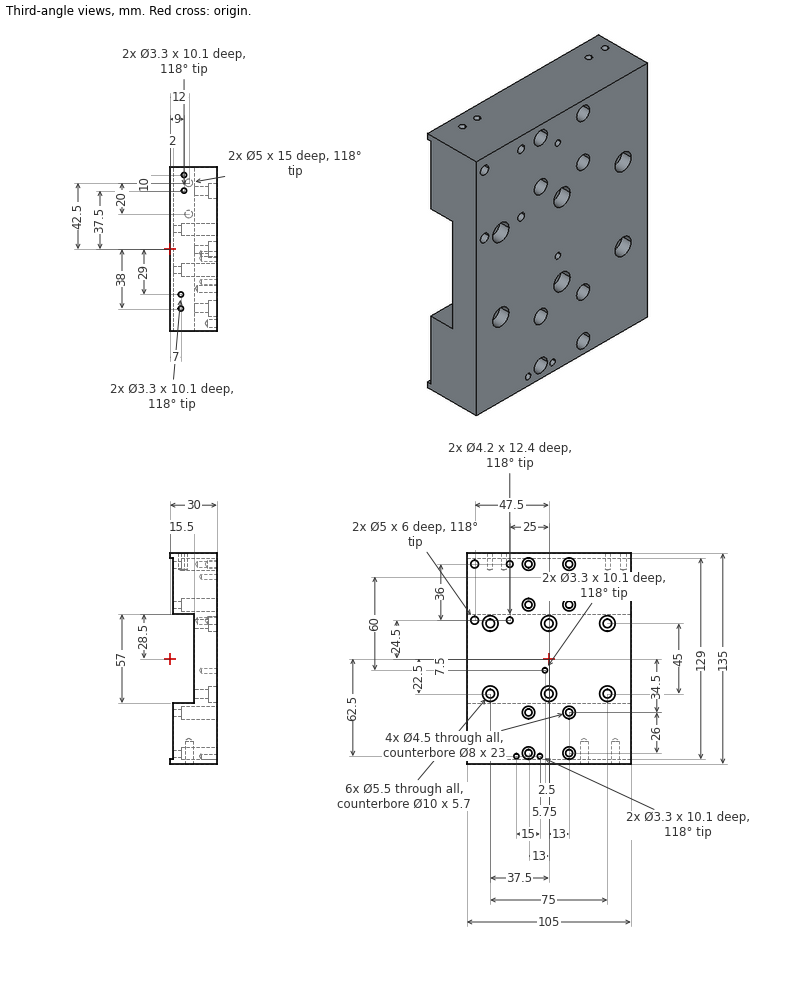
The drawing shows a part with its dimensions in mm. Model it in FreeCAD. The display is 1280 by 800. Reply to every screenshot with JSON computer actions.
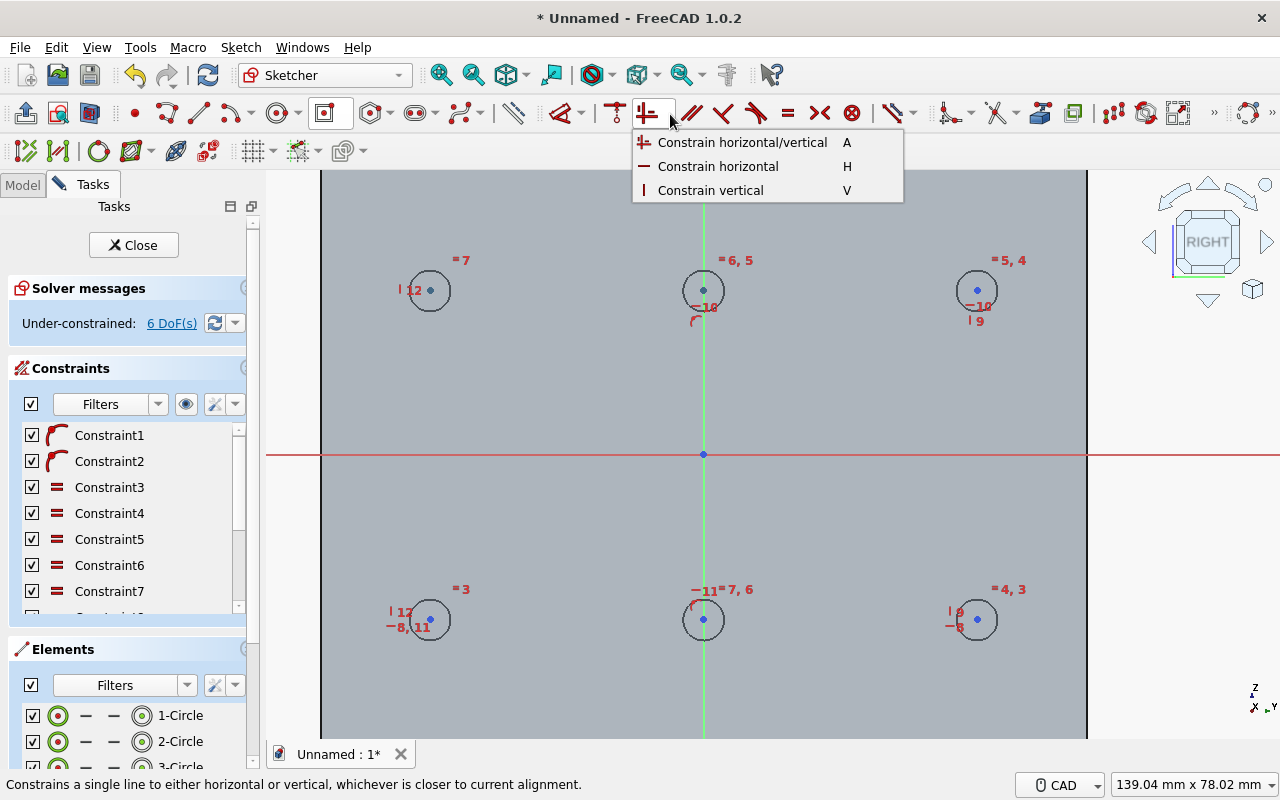
{"action": "left_click", "coordinate": [768, 166]}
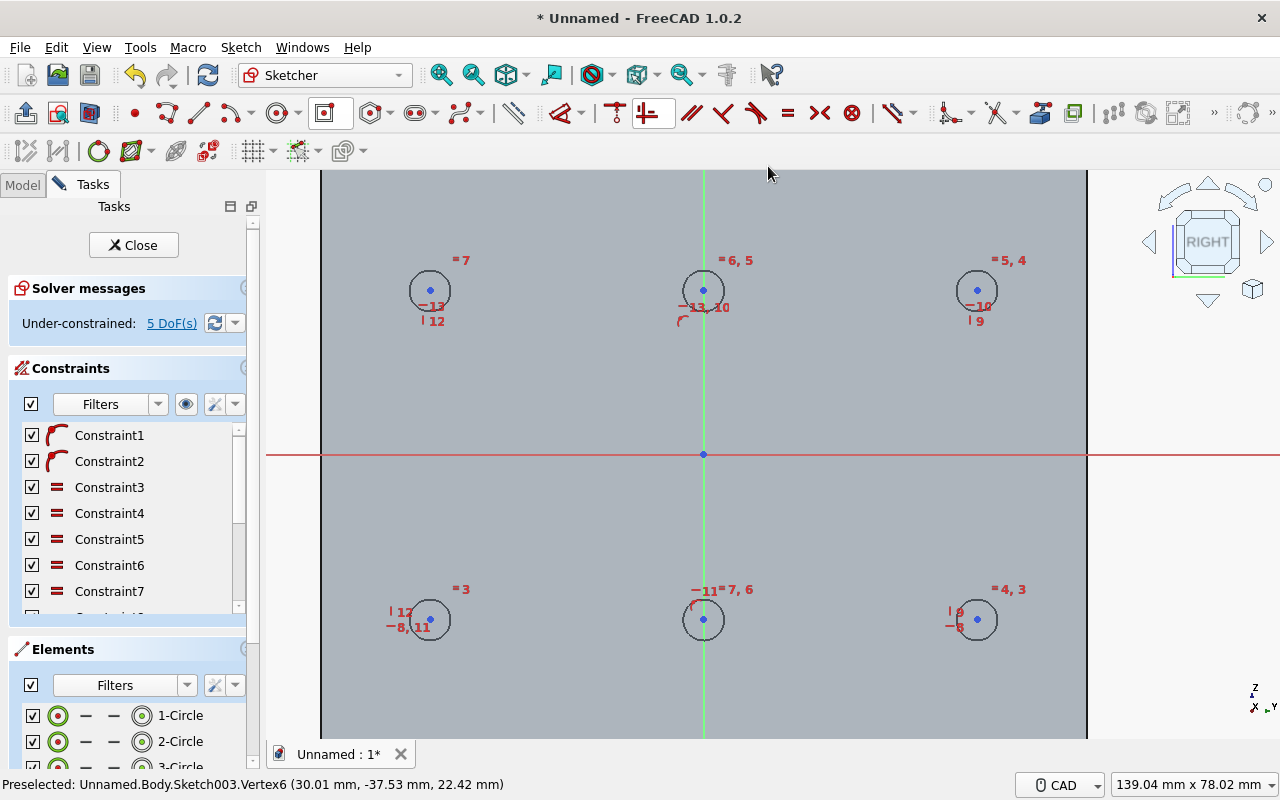
{"action": "left_click", "coordinate": [560, 114]}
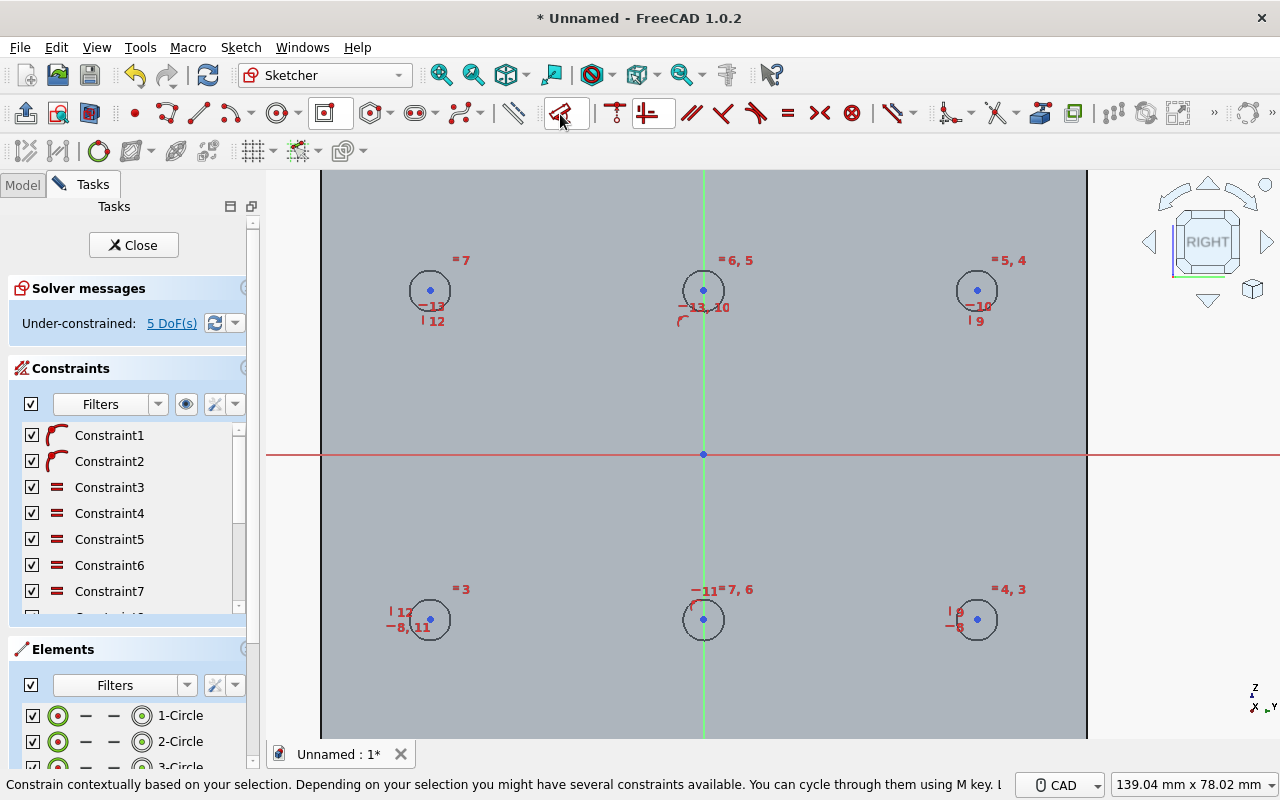
{"action": "left_click", "coordinate": [444, 605]}
{"action": "left_click", "coordinate": [466, 582]}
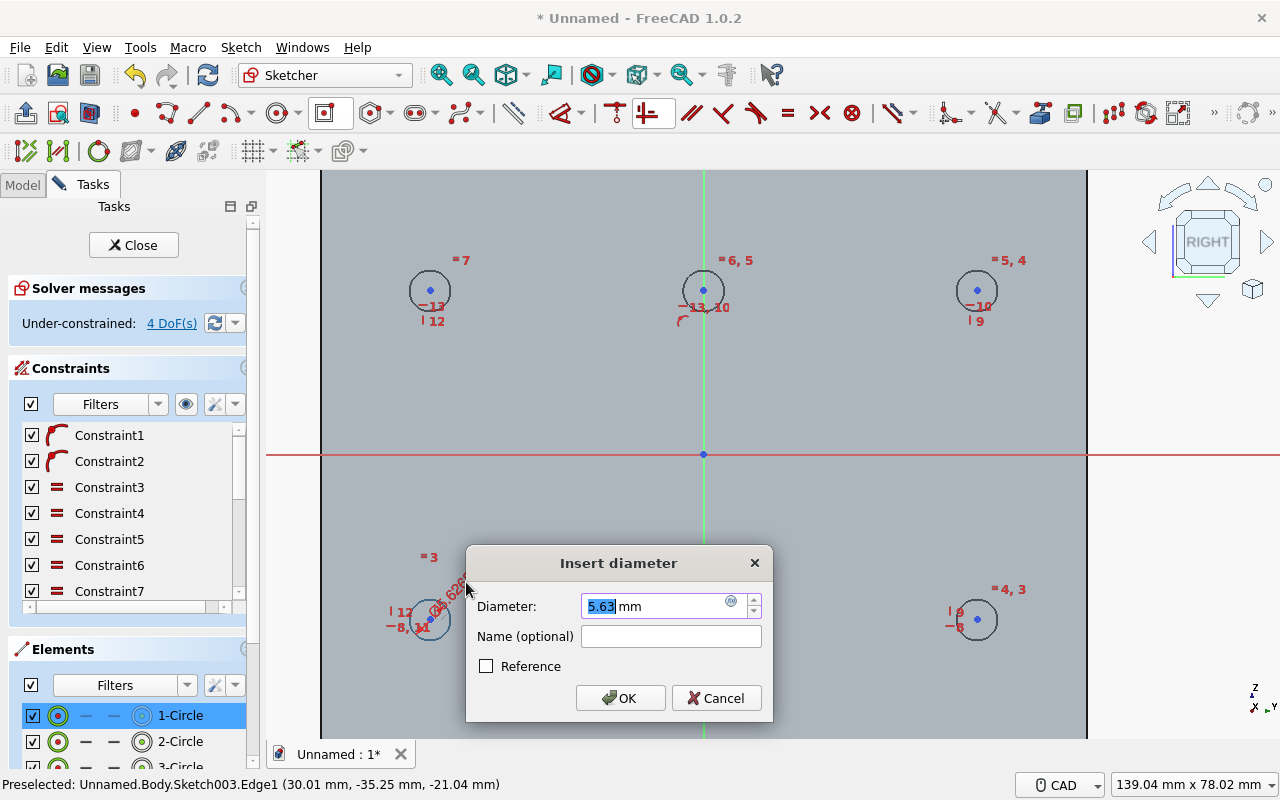
{"action": "type", "text": "5.5"}
{"action": "key", "text": "Return"}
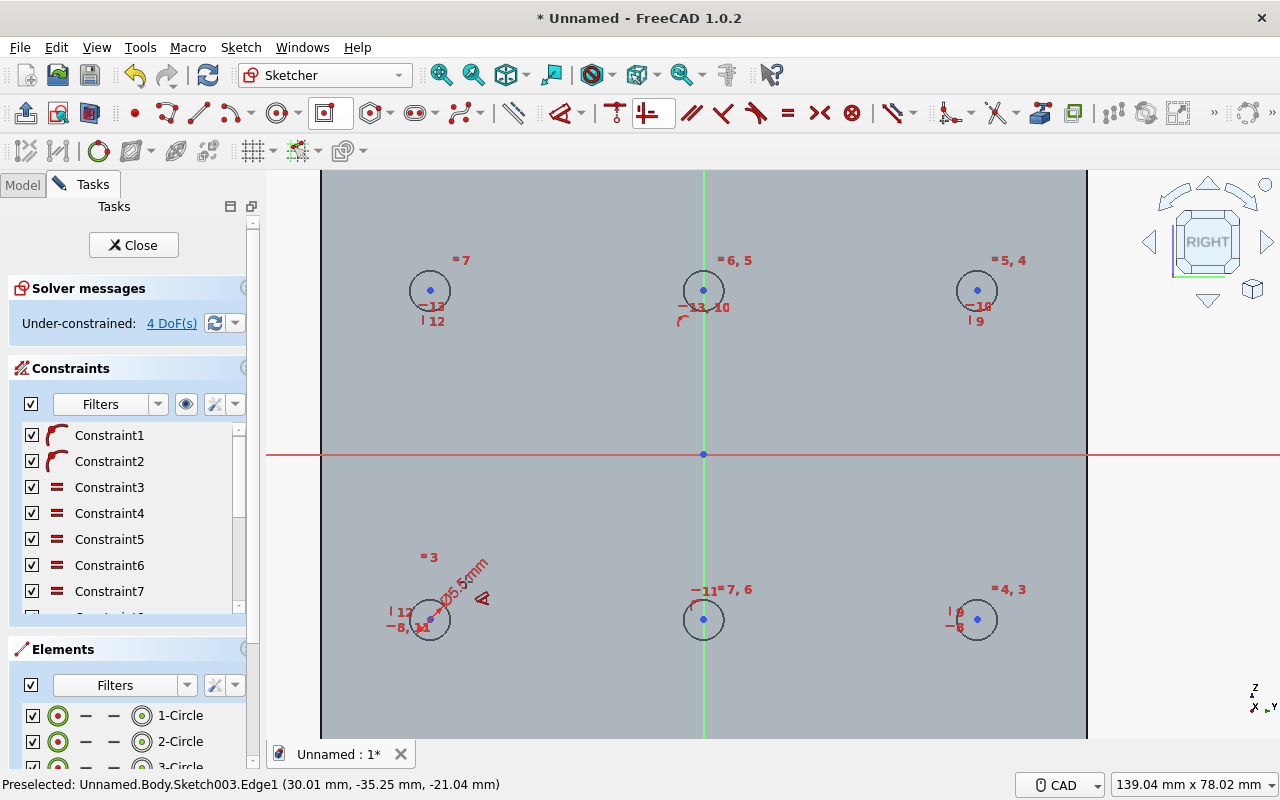
{"action": "left_click", "coordinate": [430, 620]}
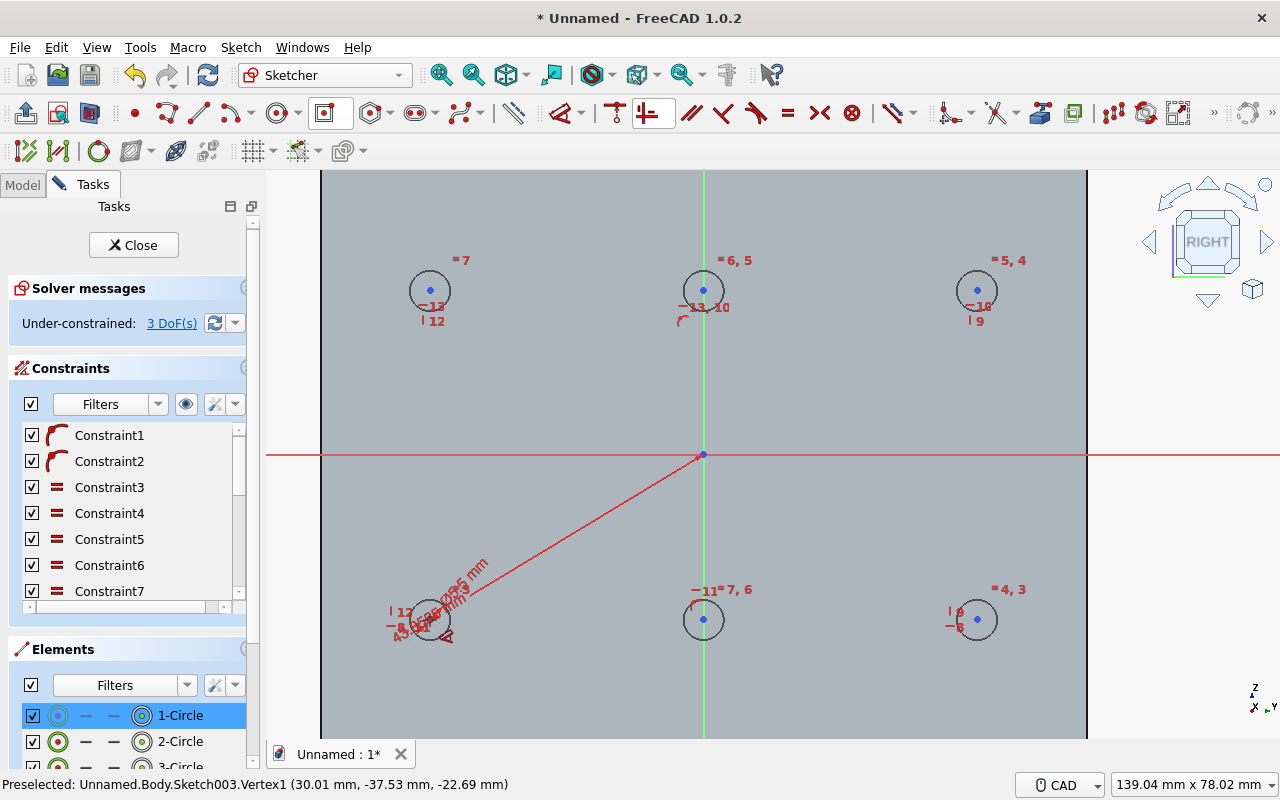
{"action": "left_click", "coordinate": [977, 620]}
{"action": "left_click", "coordinate": [578, 654]}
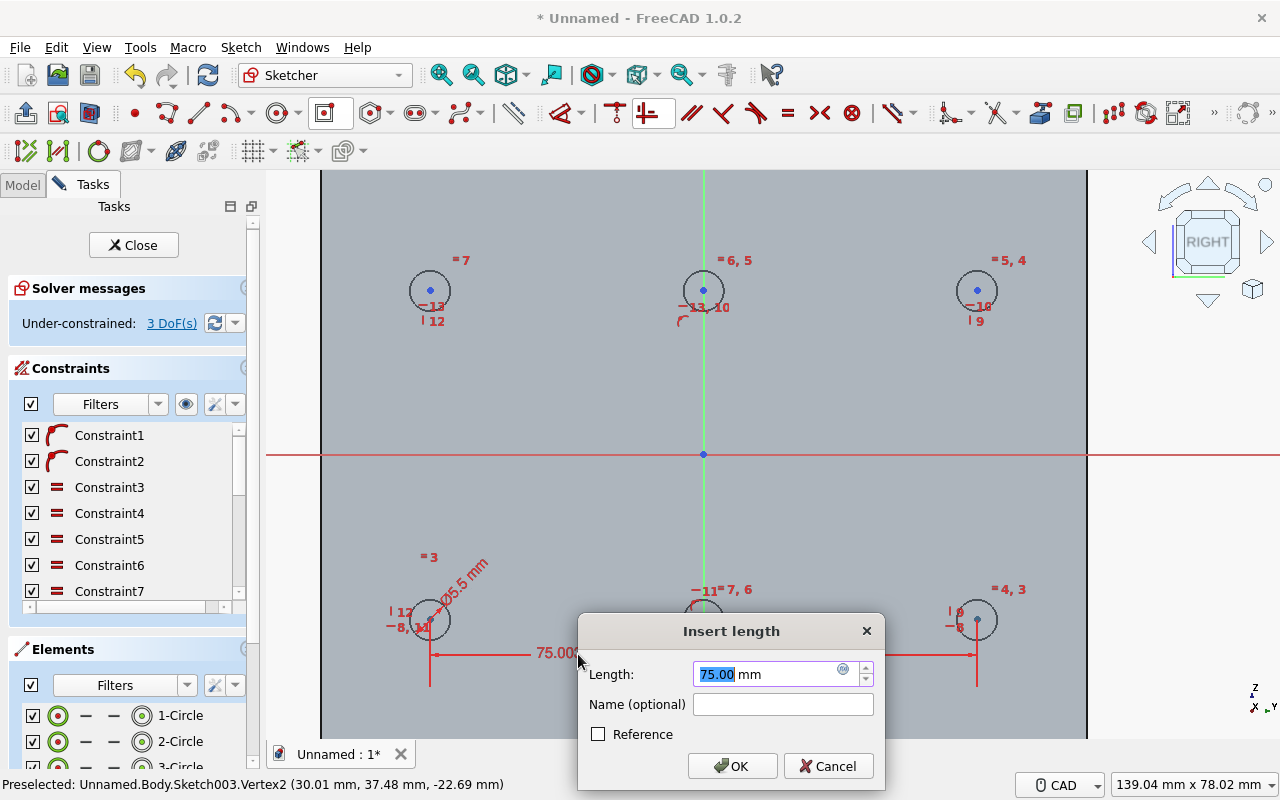
{"action": "type", "text": "75"}
{"action": "key", "text": "Return"}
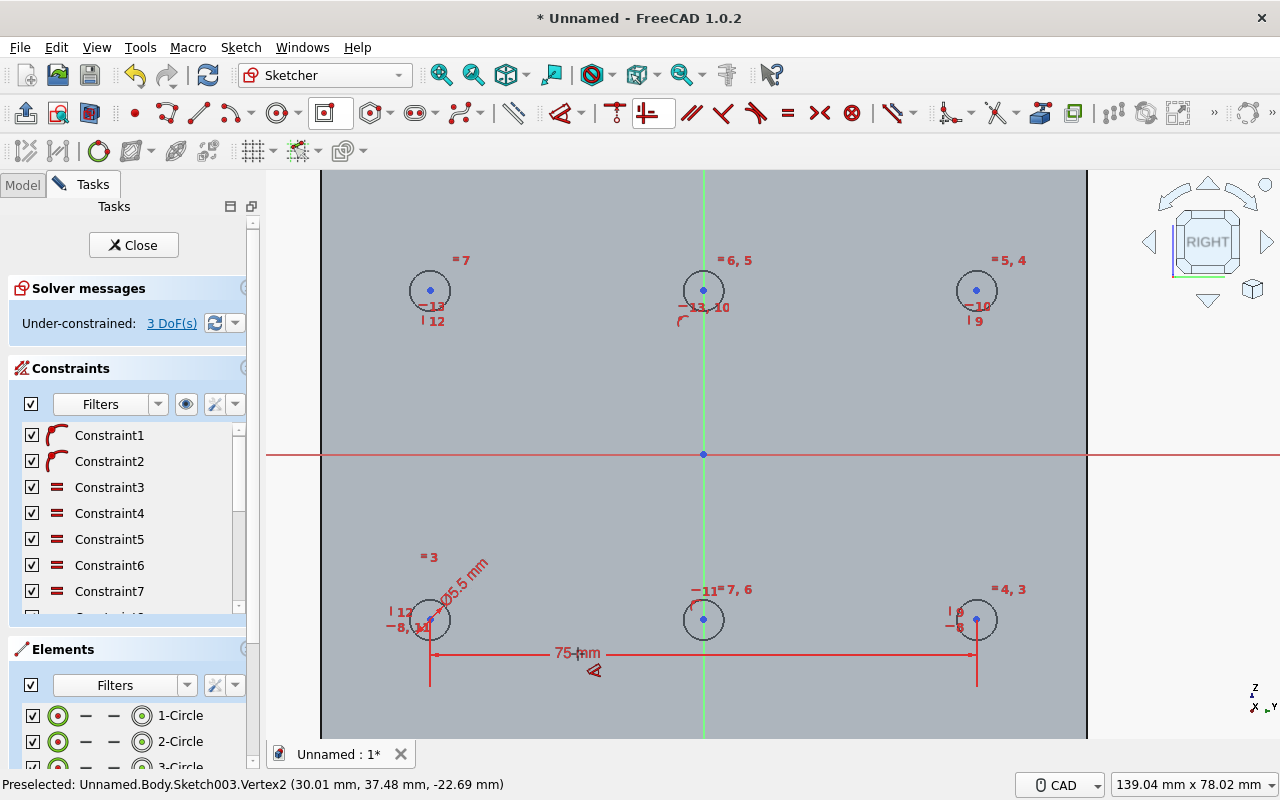
{"action": "left_click", "coordinate": [977, 620]}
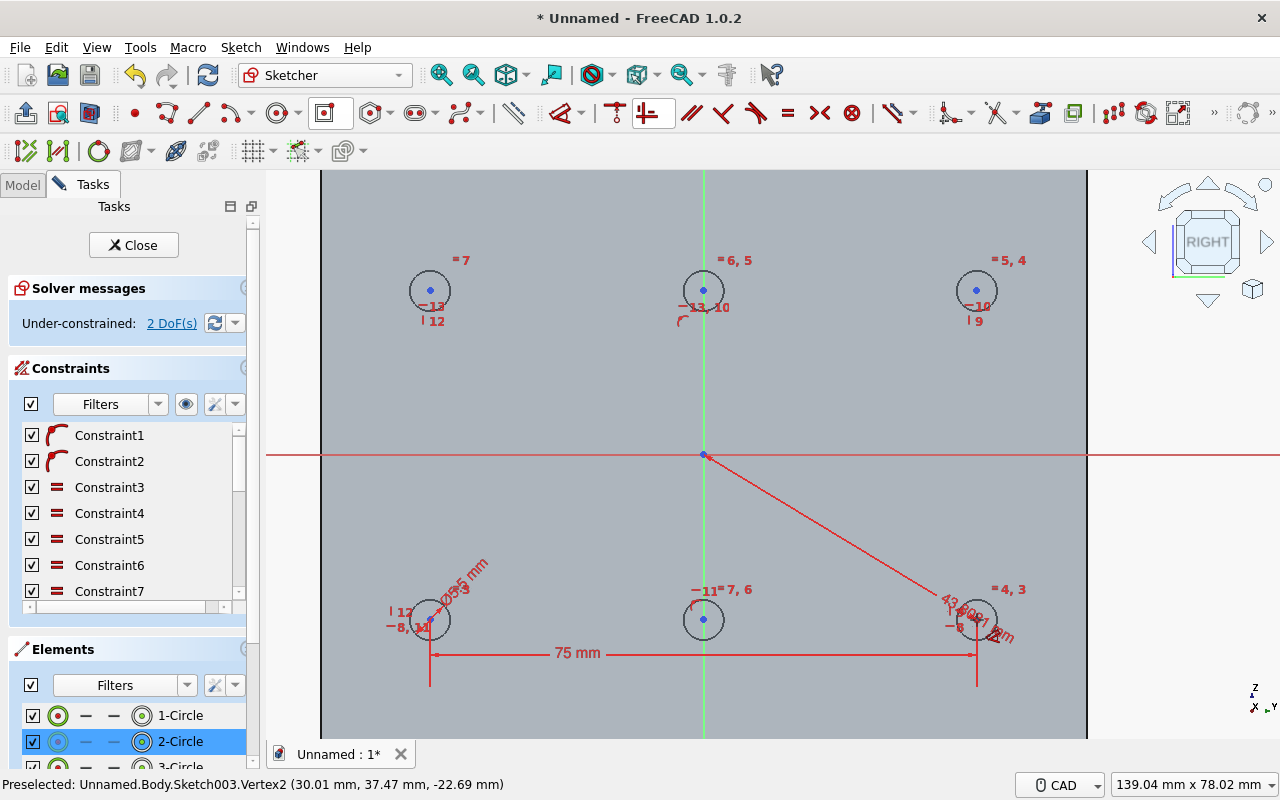
{"action": "left_click", "coordinate": [977, 291]}
{"action": "left_click", "coordinate": [1011, 380]}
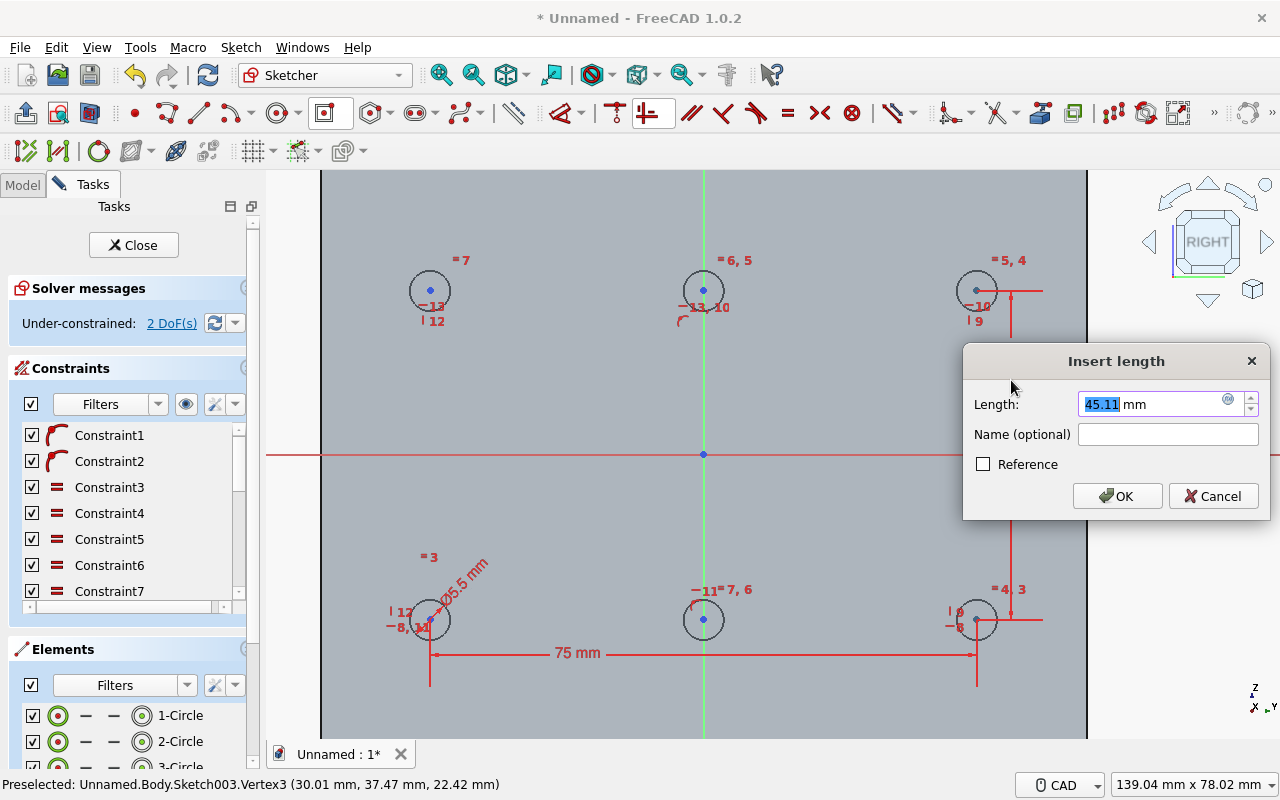
{"action": "type", "text": "45"}
{"action": "key", "text": "Return"}